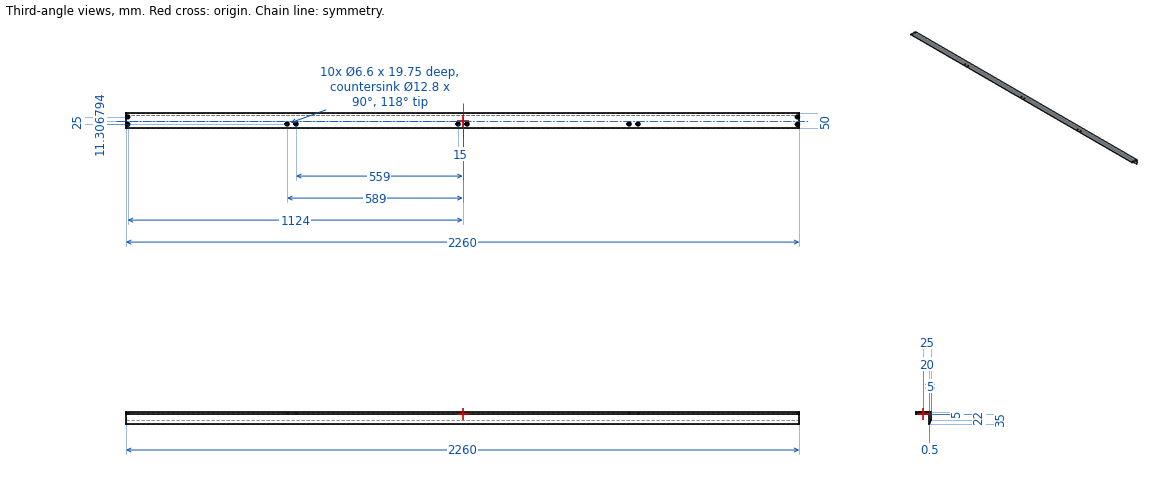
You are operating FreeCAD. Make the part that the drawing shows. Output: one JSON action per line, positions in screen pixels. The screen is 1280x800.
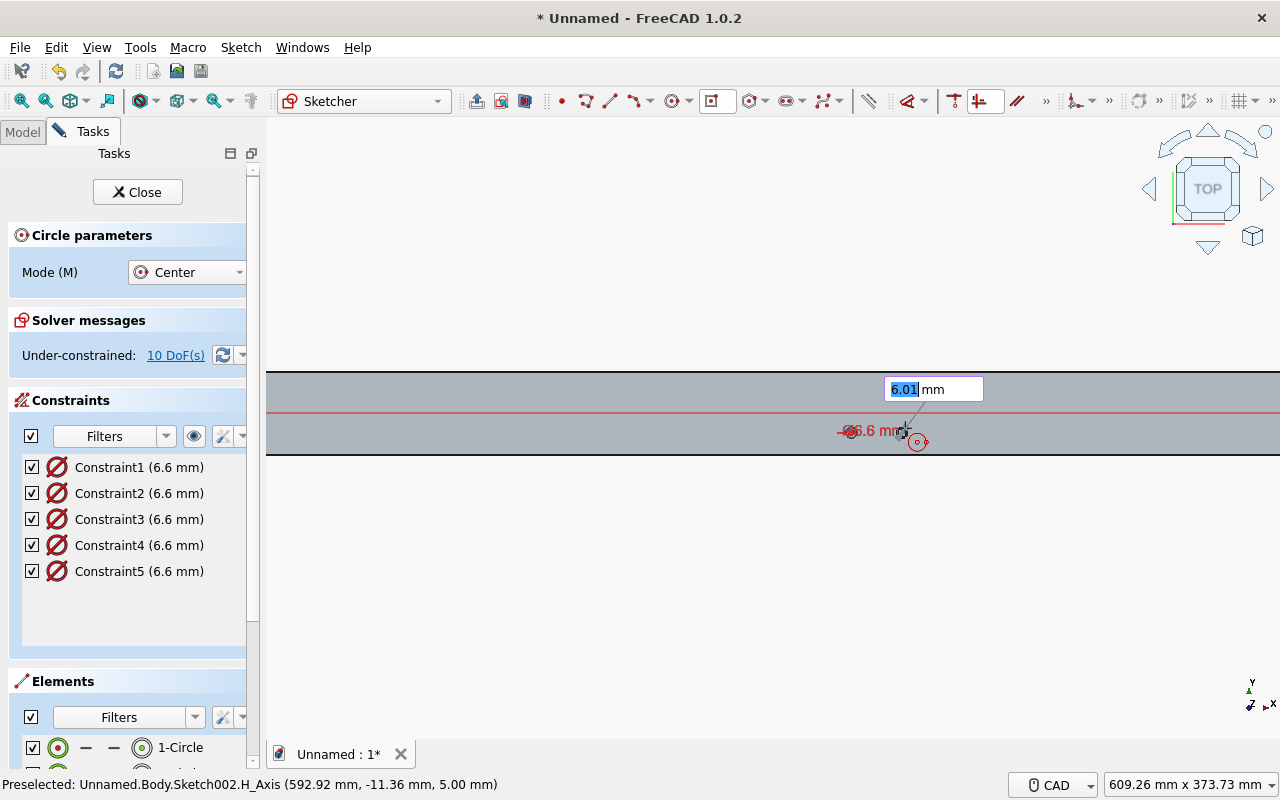
{"action": "type", "text": "6.6"}
{"action": "key", "text": "Return"}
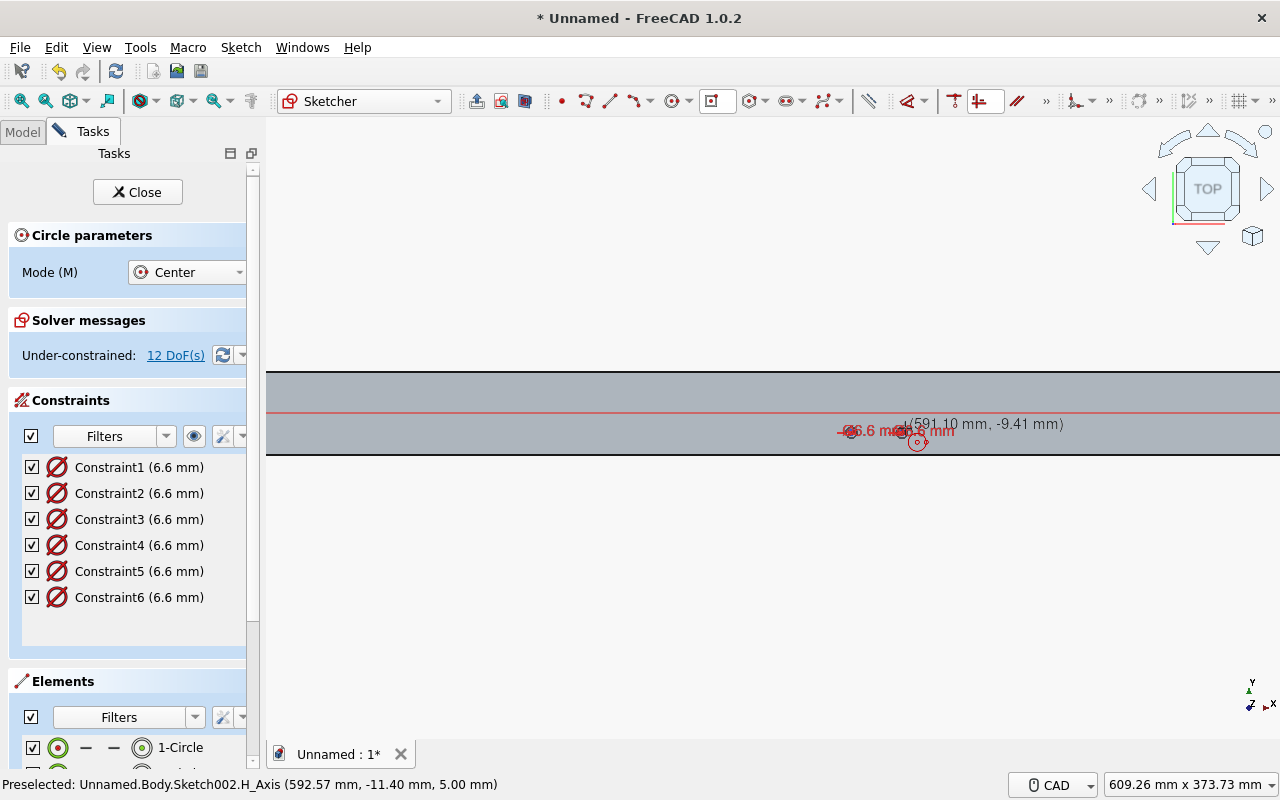
{"action": "scroll", "coordinate": [860, 431], "scroll_direction": "down", "scroll_amount": 9}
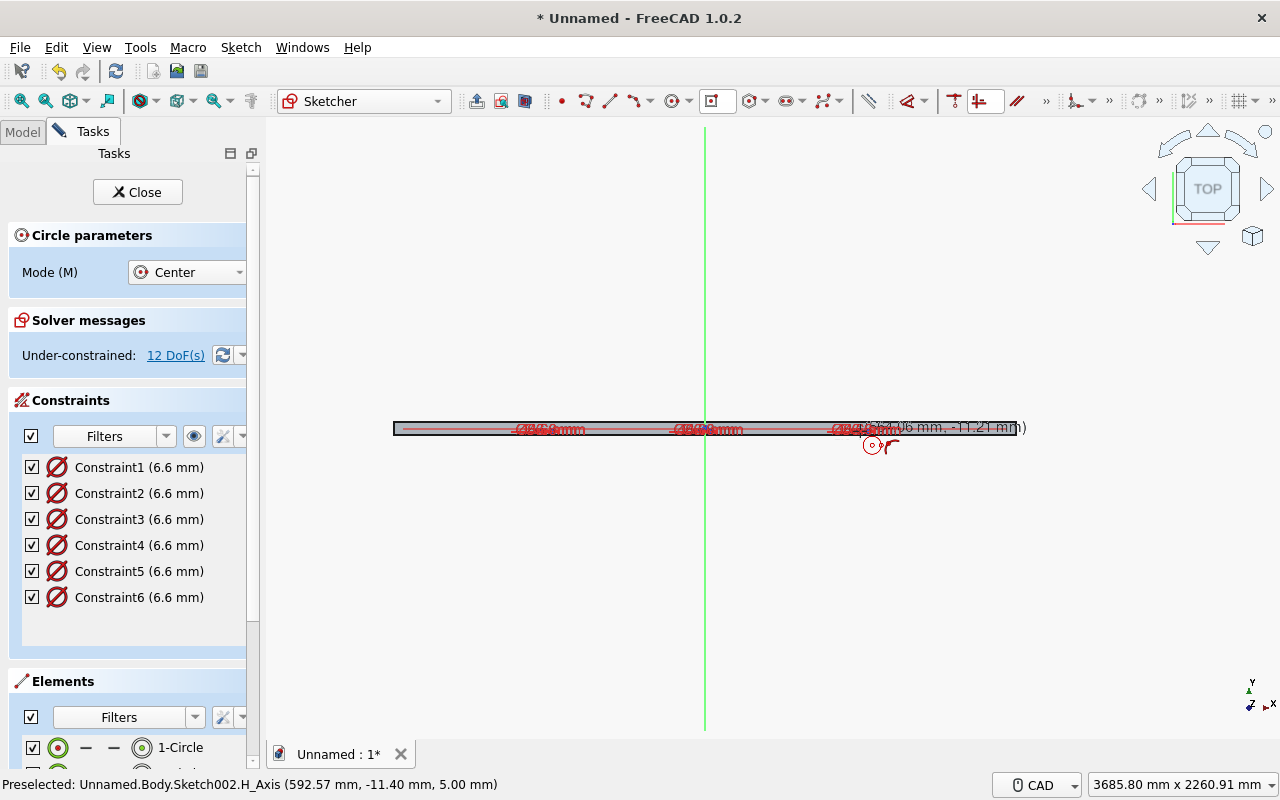
{"action": "scroll", "coordinate": [396, 432], "scroll_direction": "up", "scroll_amount": 17}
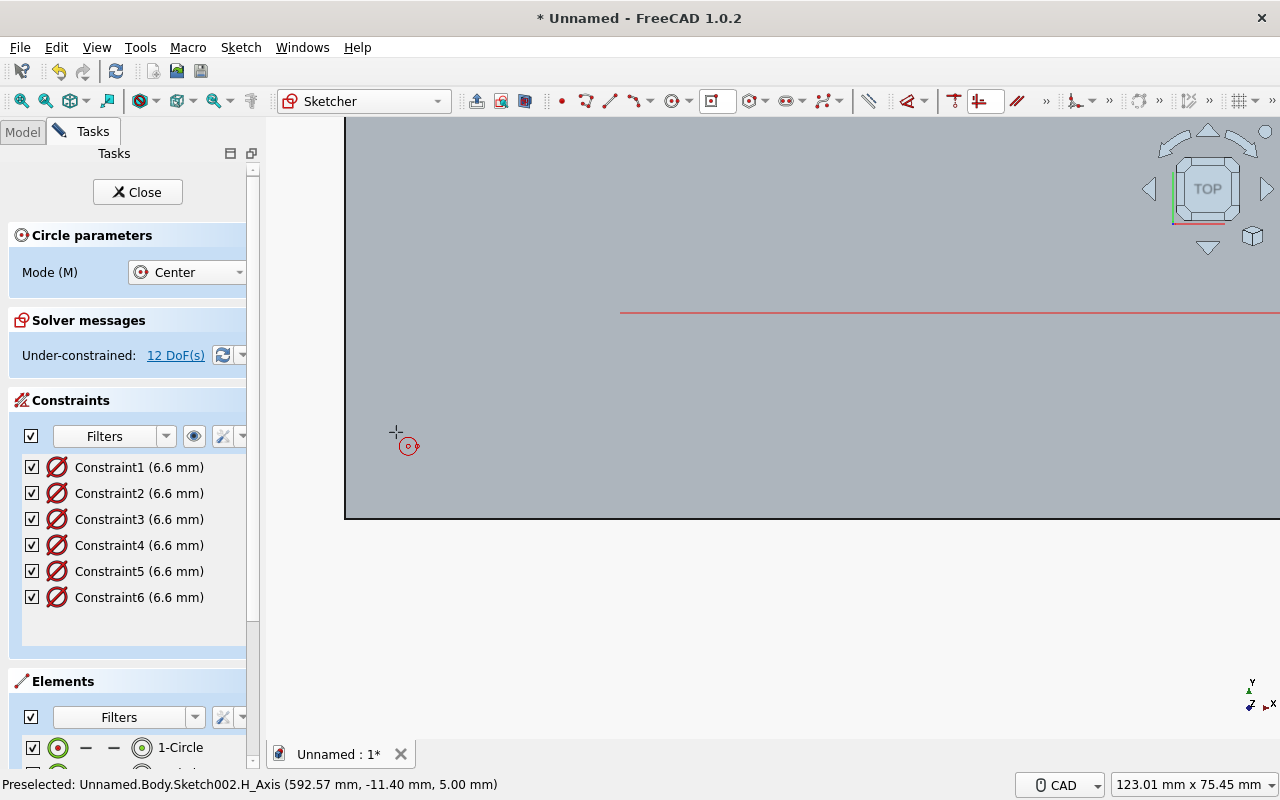
{"action": "scroll", "coordinate": [324, 433], "scroll_direction": "down", "scroll_amount": 16}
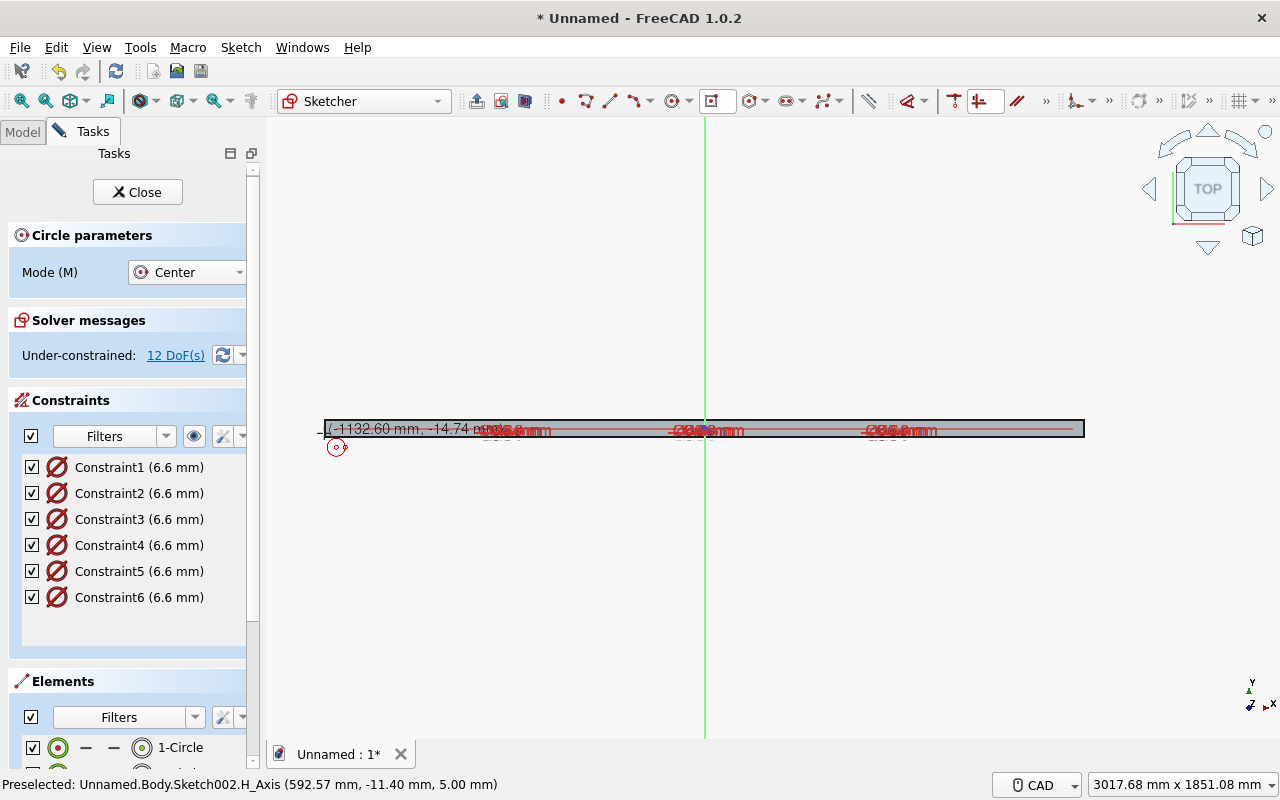
{"action": "scroll", "coordinate": [327, 433], "scroll_direction": "up", "scroll_amount": 7}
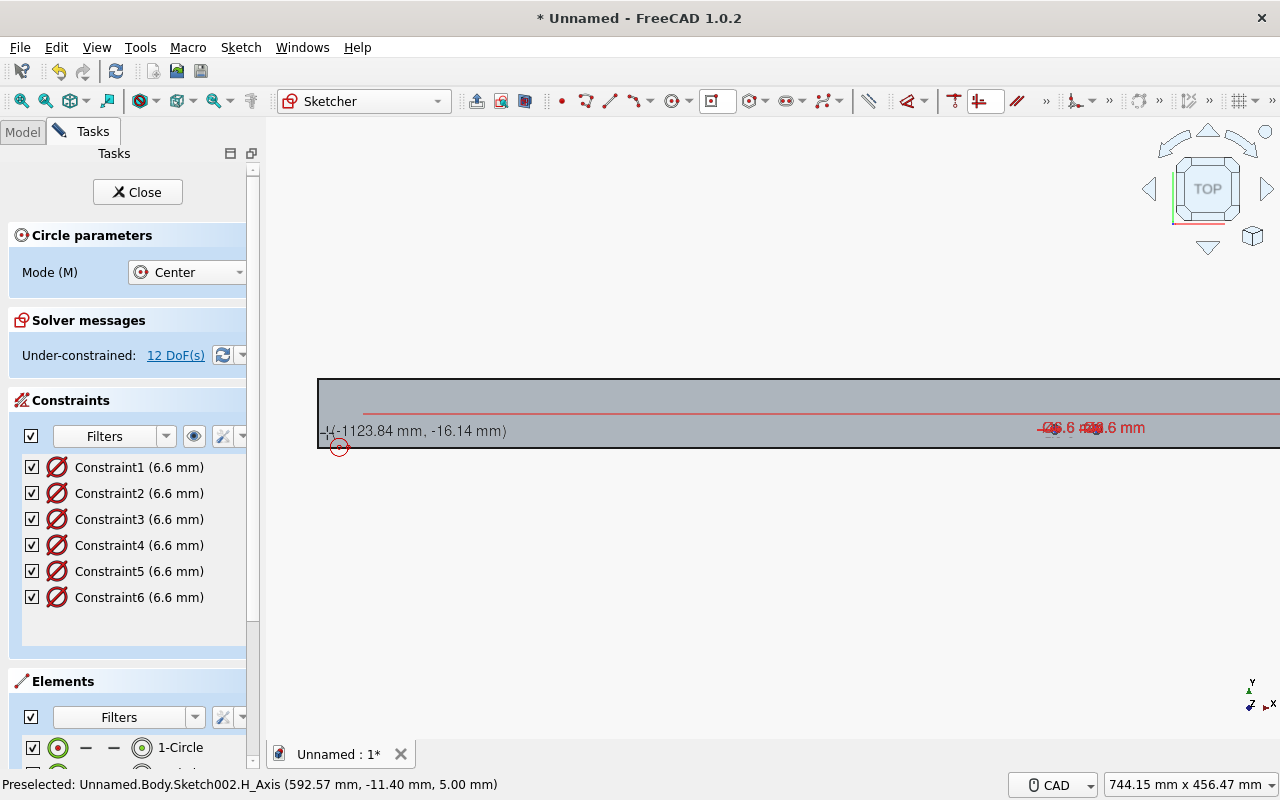
{"action": "left_click", "coordinate": [327, 431]}
{"action": "mouse_move", "coordinate": [330, 434]}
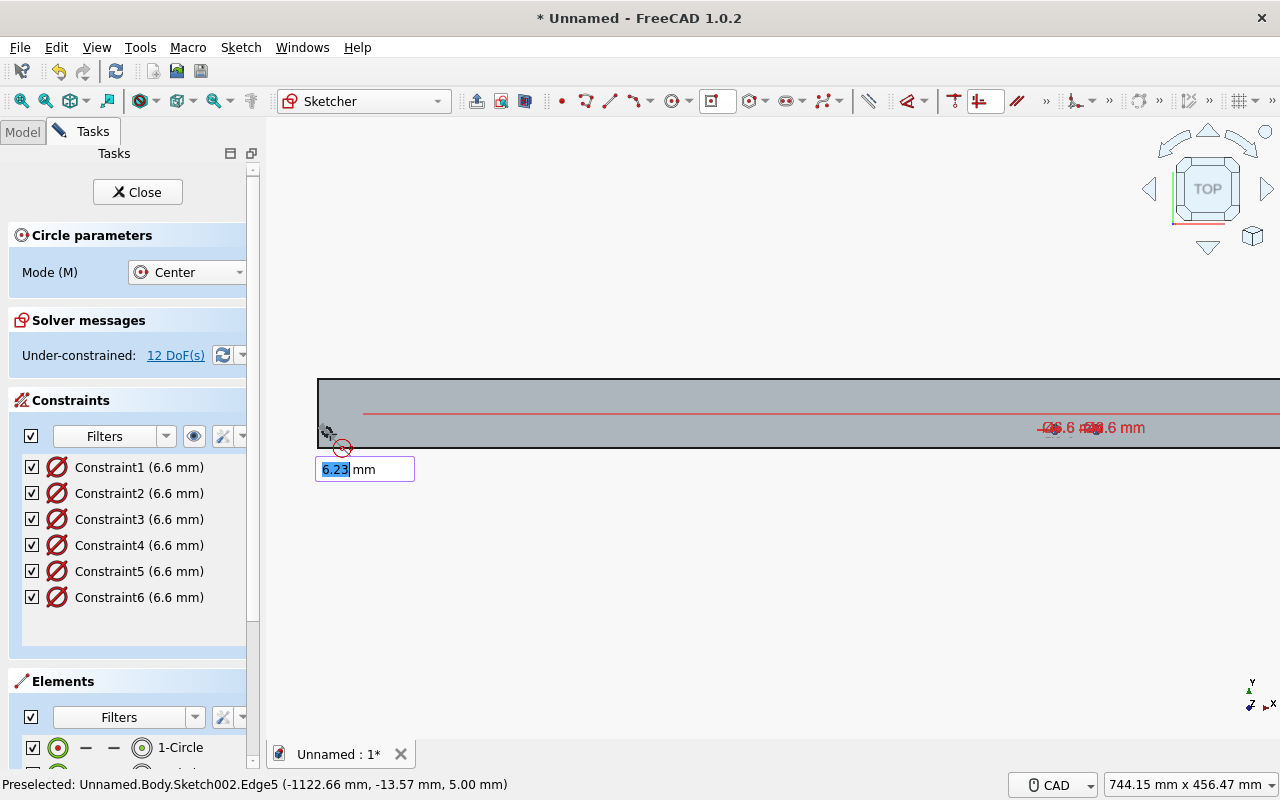
{"action": "type", "text": "6.6"}
{"action": "key", "text": "Return"}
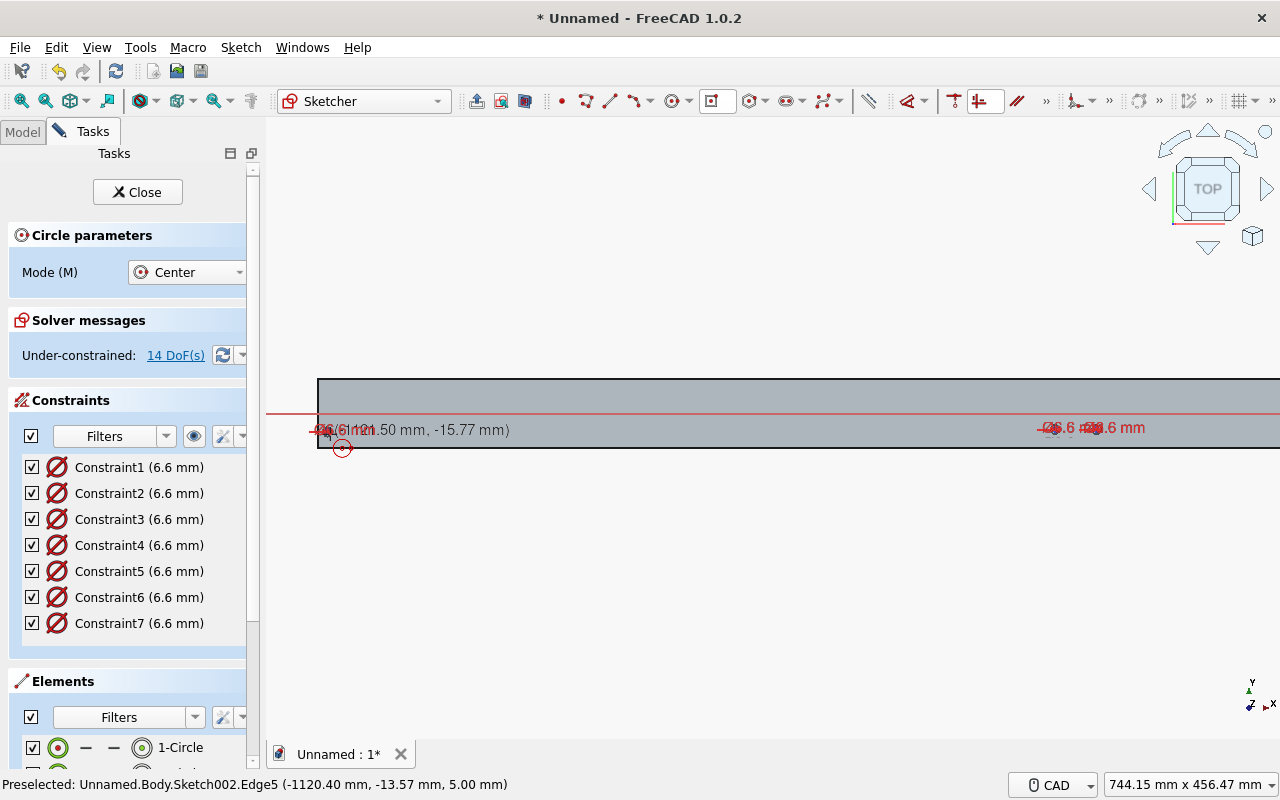
{"action": "scroll", "coordinate": [327, 396], "scroll_direction": "up", "scroll_amount": 9}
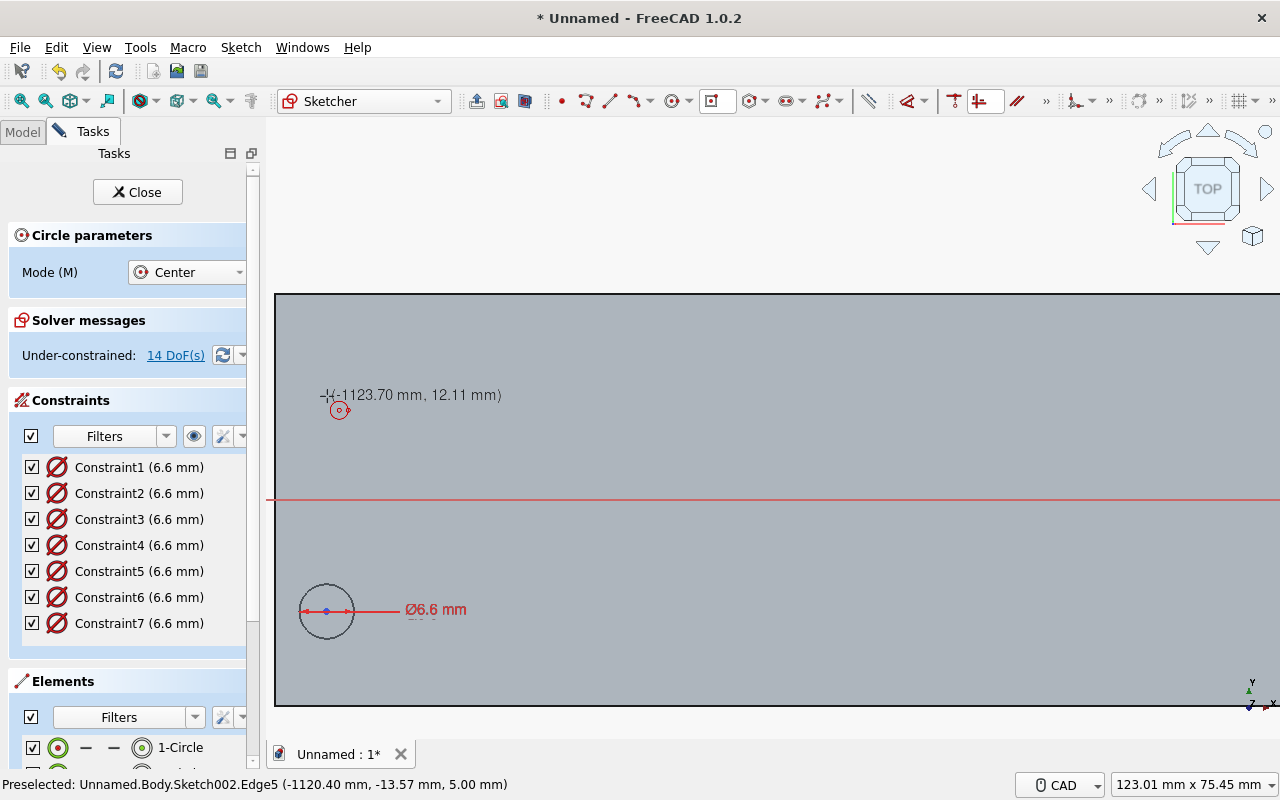
{"action": "scroll", "coordinate": [327, 425], "scroll_direction": "down", "scroll_amount": 16}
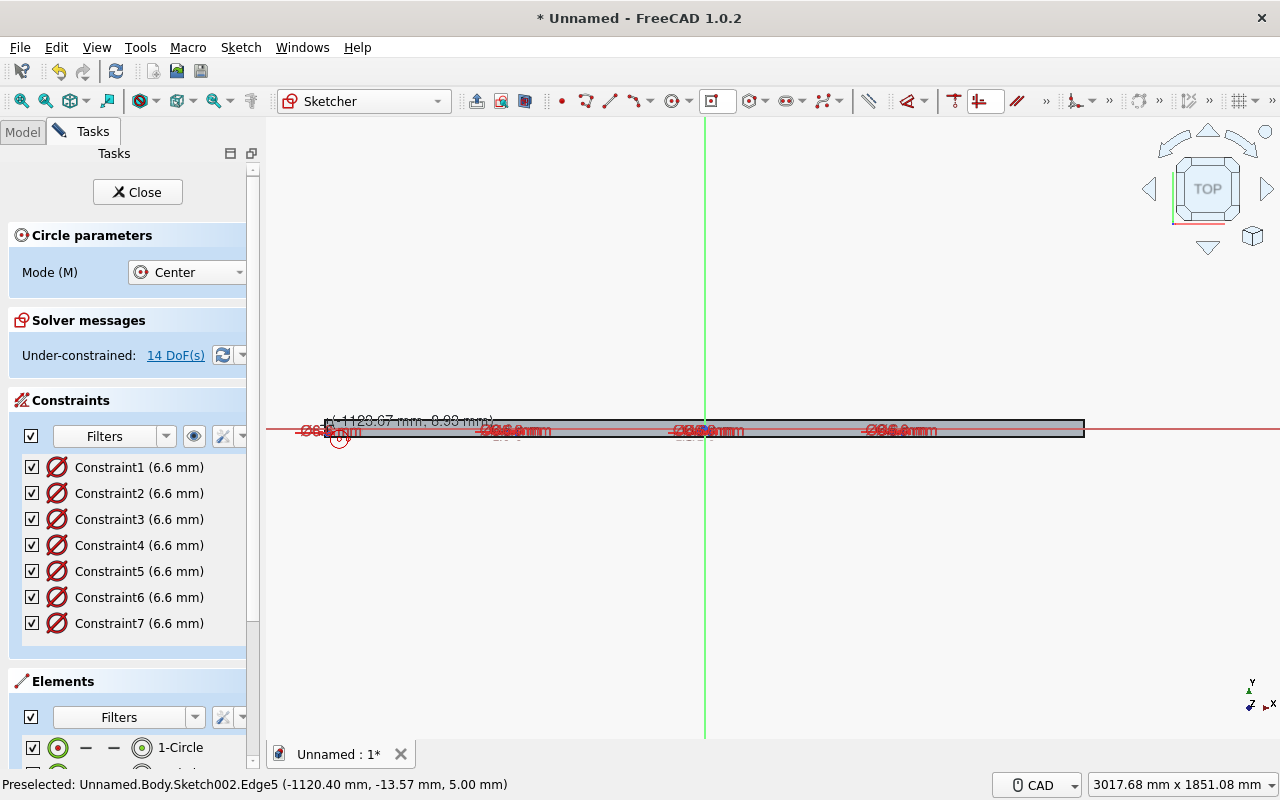
{"action": "scroll", "coordinate": [327, 424], "scroll_direction": "up", "scroll_amount": 7}